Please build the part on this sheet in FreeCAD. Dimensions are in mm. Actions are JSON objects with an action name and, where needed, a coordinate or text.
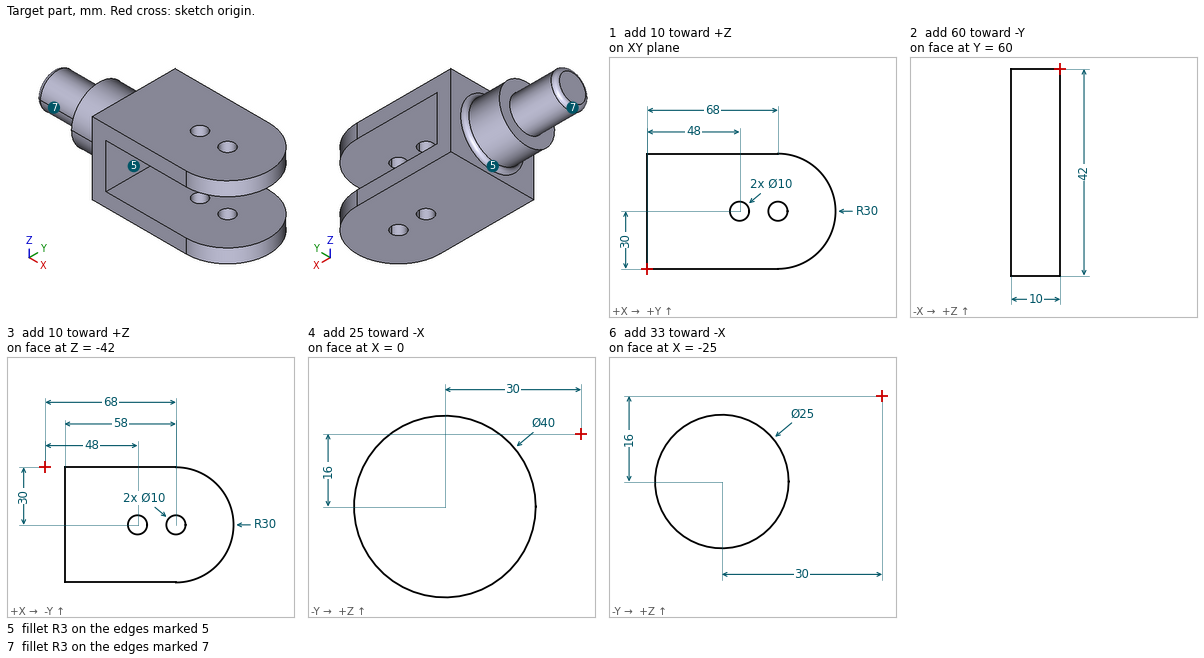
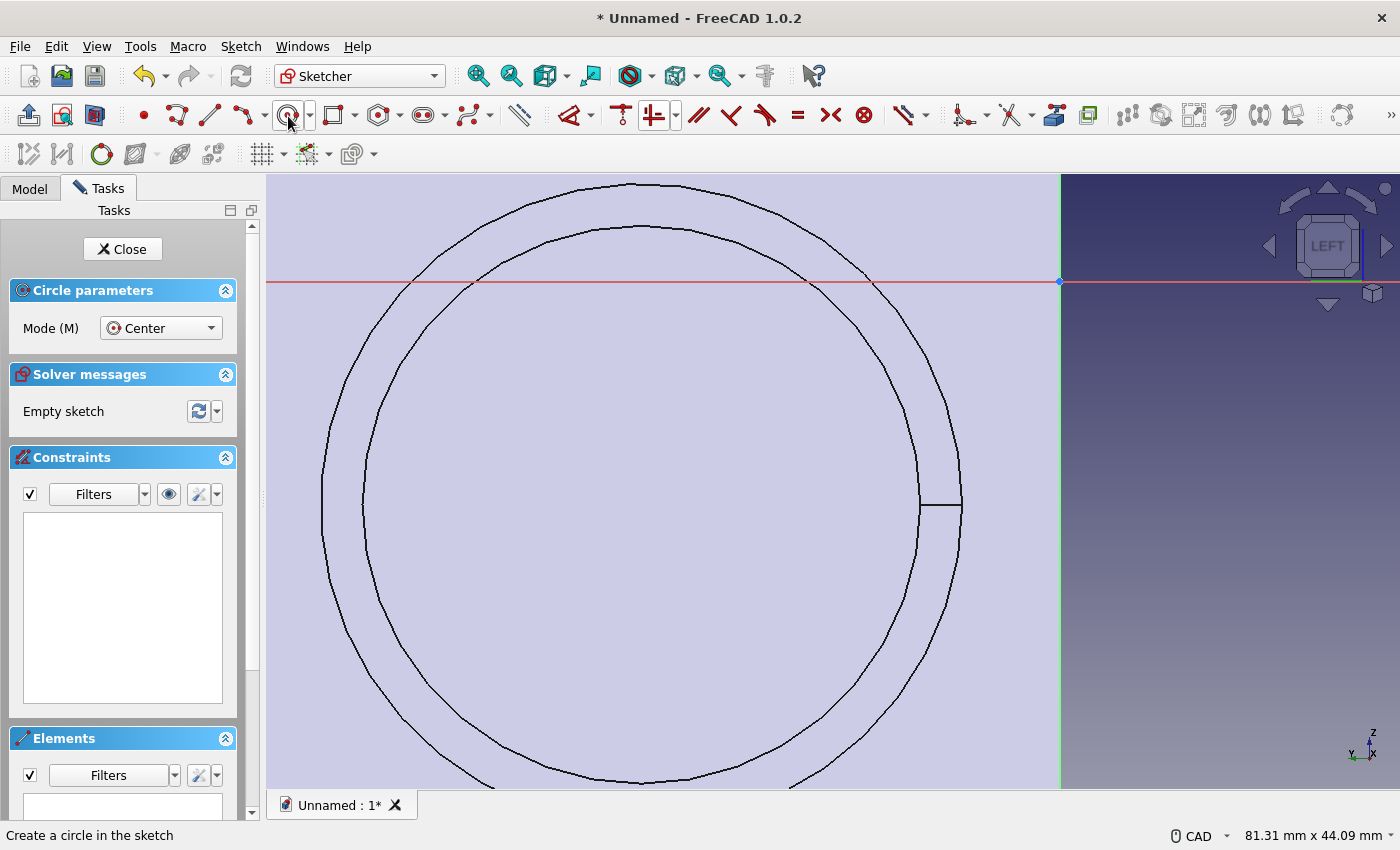
{"action": "left_click", "coordinate": [641, 505]}
{"action": "mouse_move", "coordinate": [765, 381]}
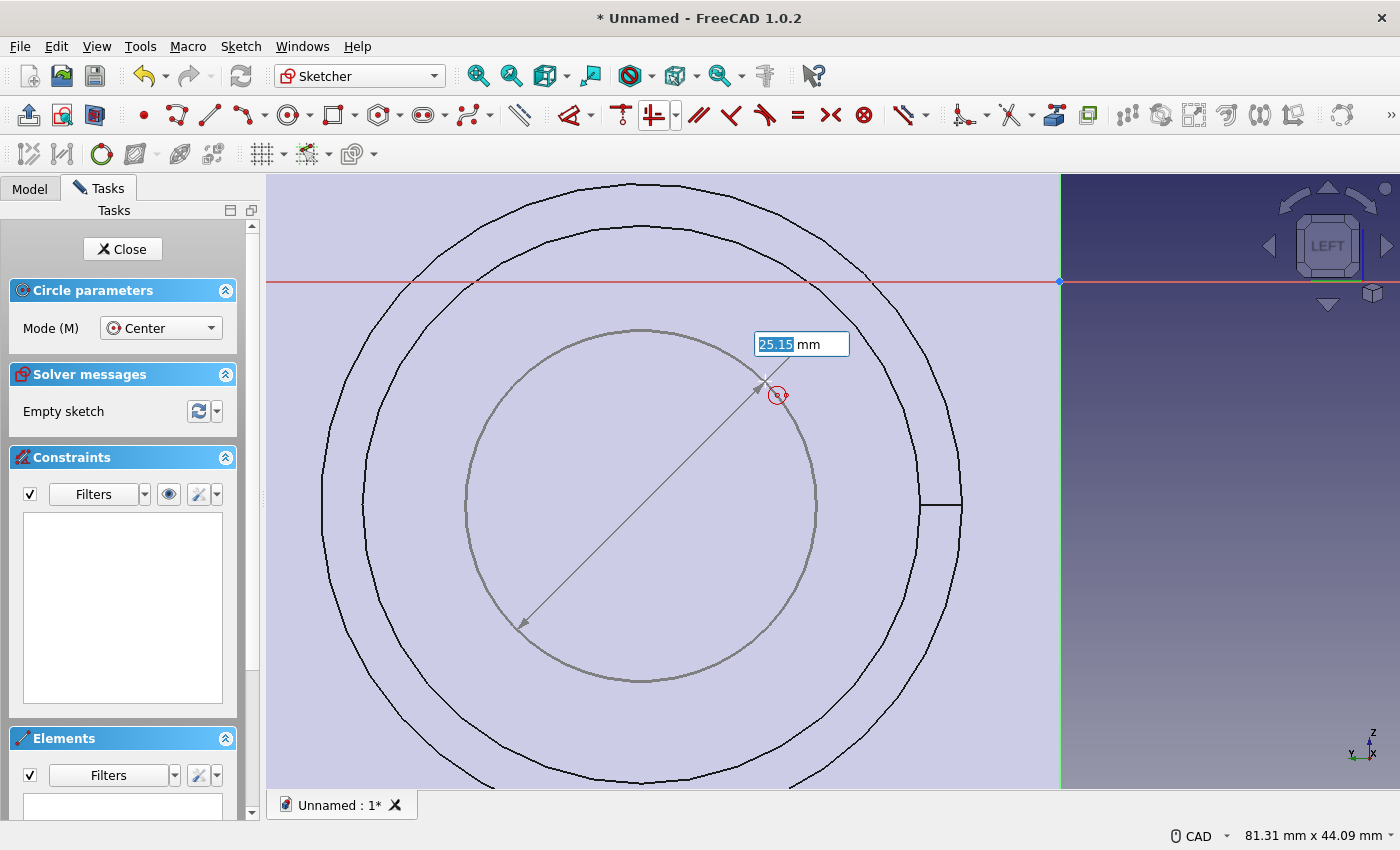
{"action": "type", "text": "25"}
{"action": "key", "text": "Return"}
{"action": "key", "text": "Escape"}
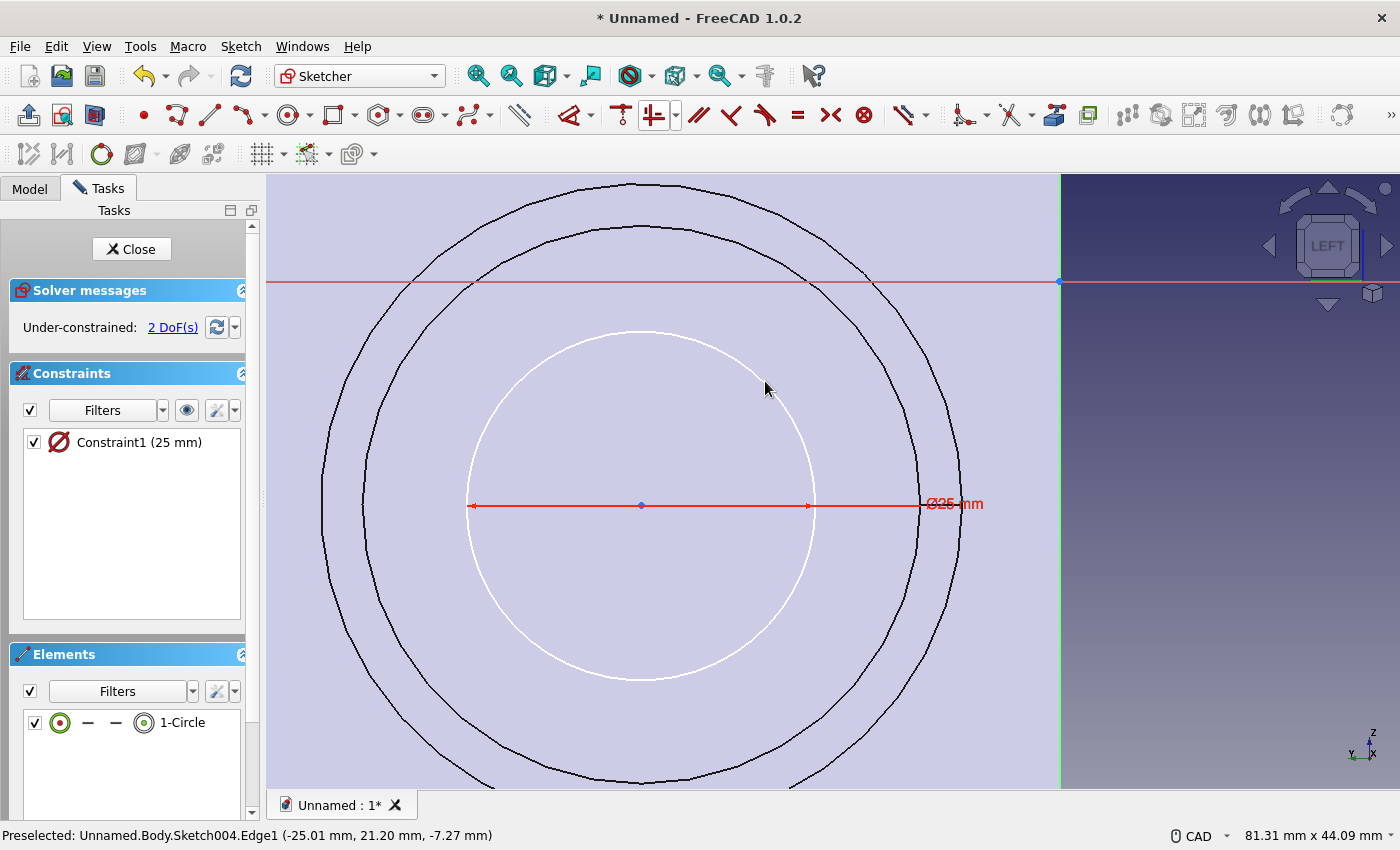
{"action": "left_click", "coordinate": [568, 116]}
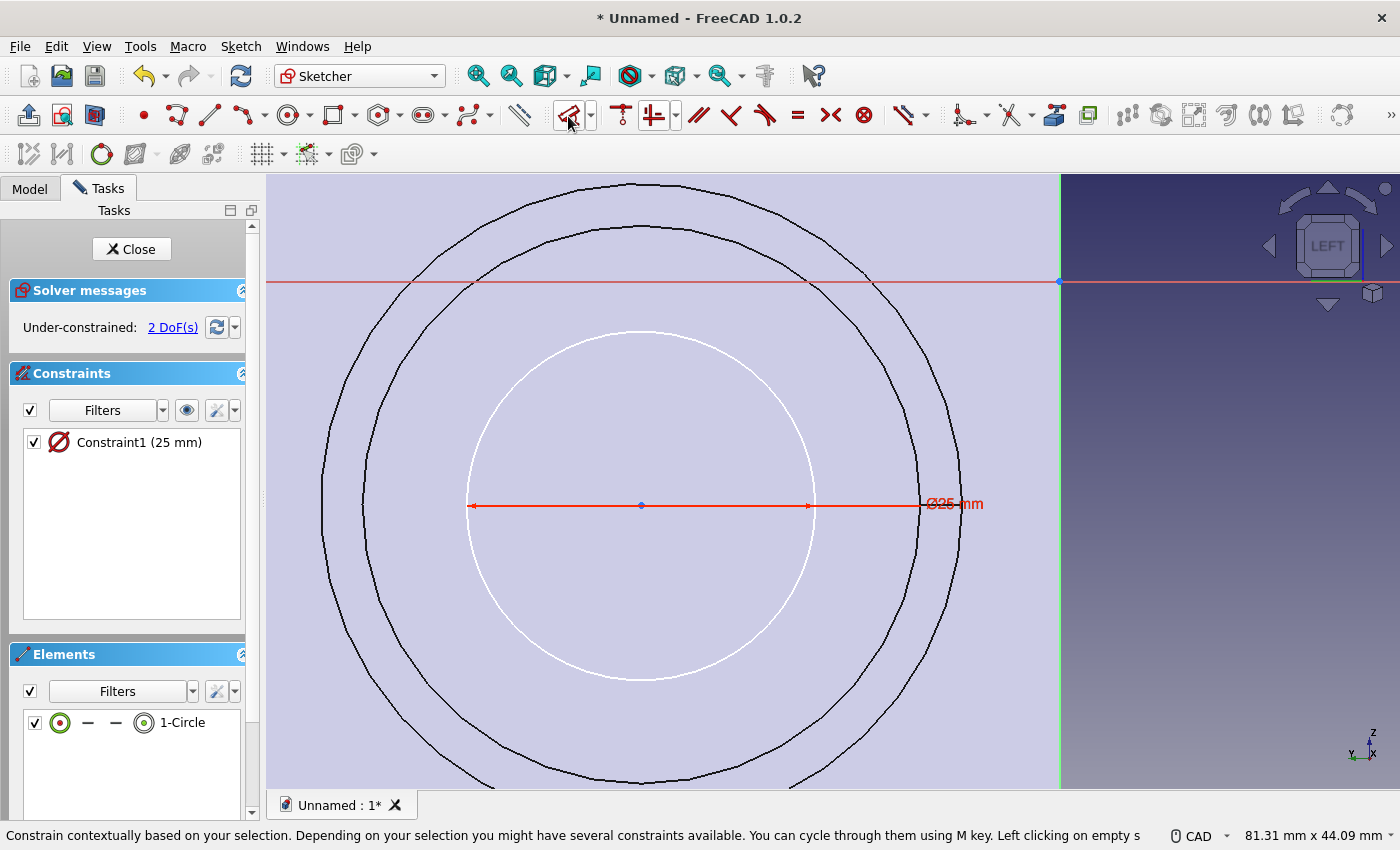
{"action": "left_click", "coordinate": [641, 506]}
{"action": "left_click", "coordinate": [850, 248]}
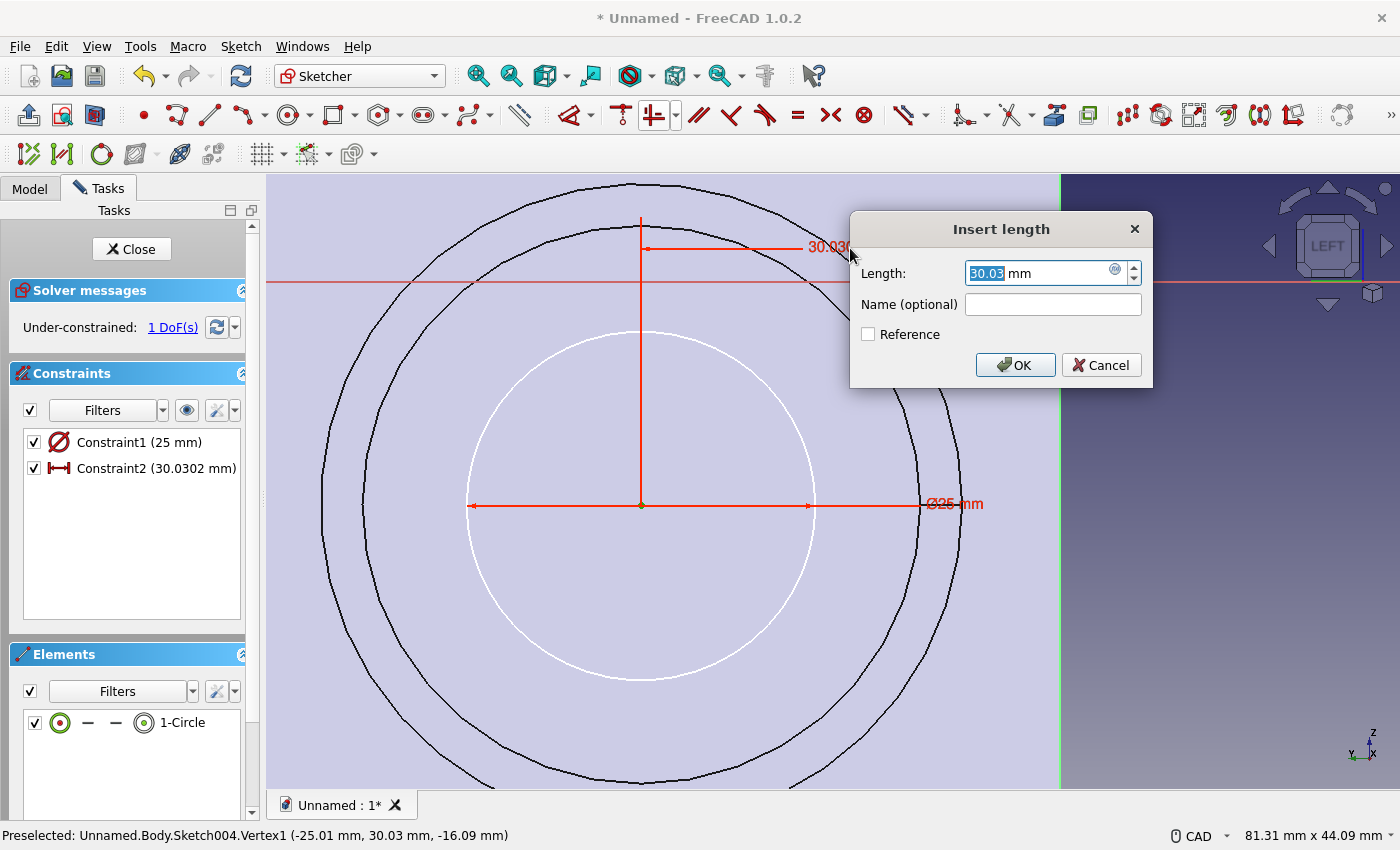
{"action": "type", "text": "30"}
{"action": "key", "text": "Return"}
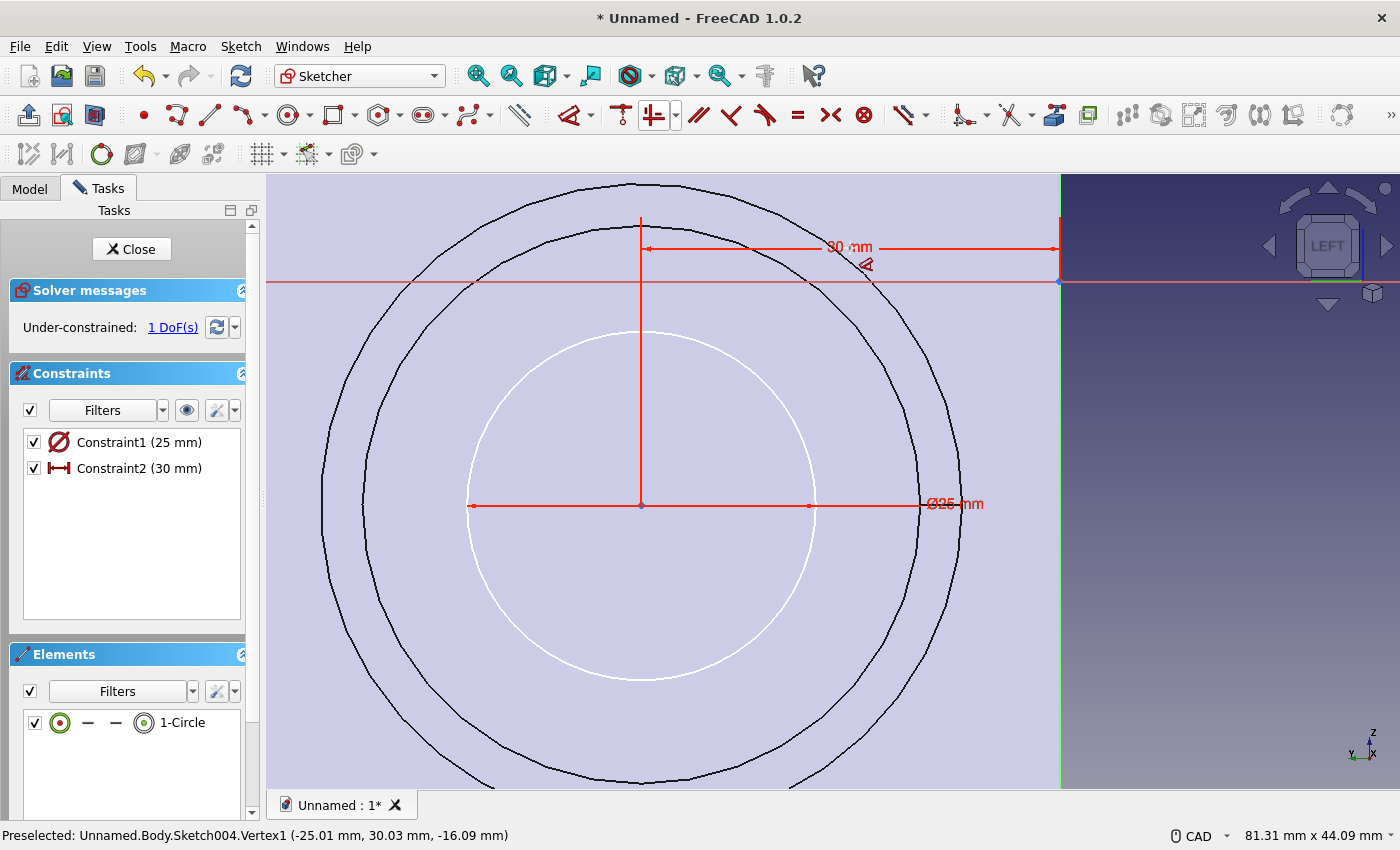
{"action": "left_click", "coordinate": [641, 506]}
{"action": "left_click", "coordinate": [1094, 394]}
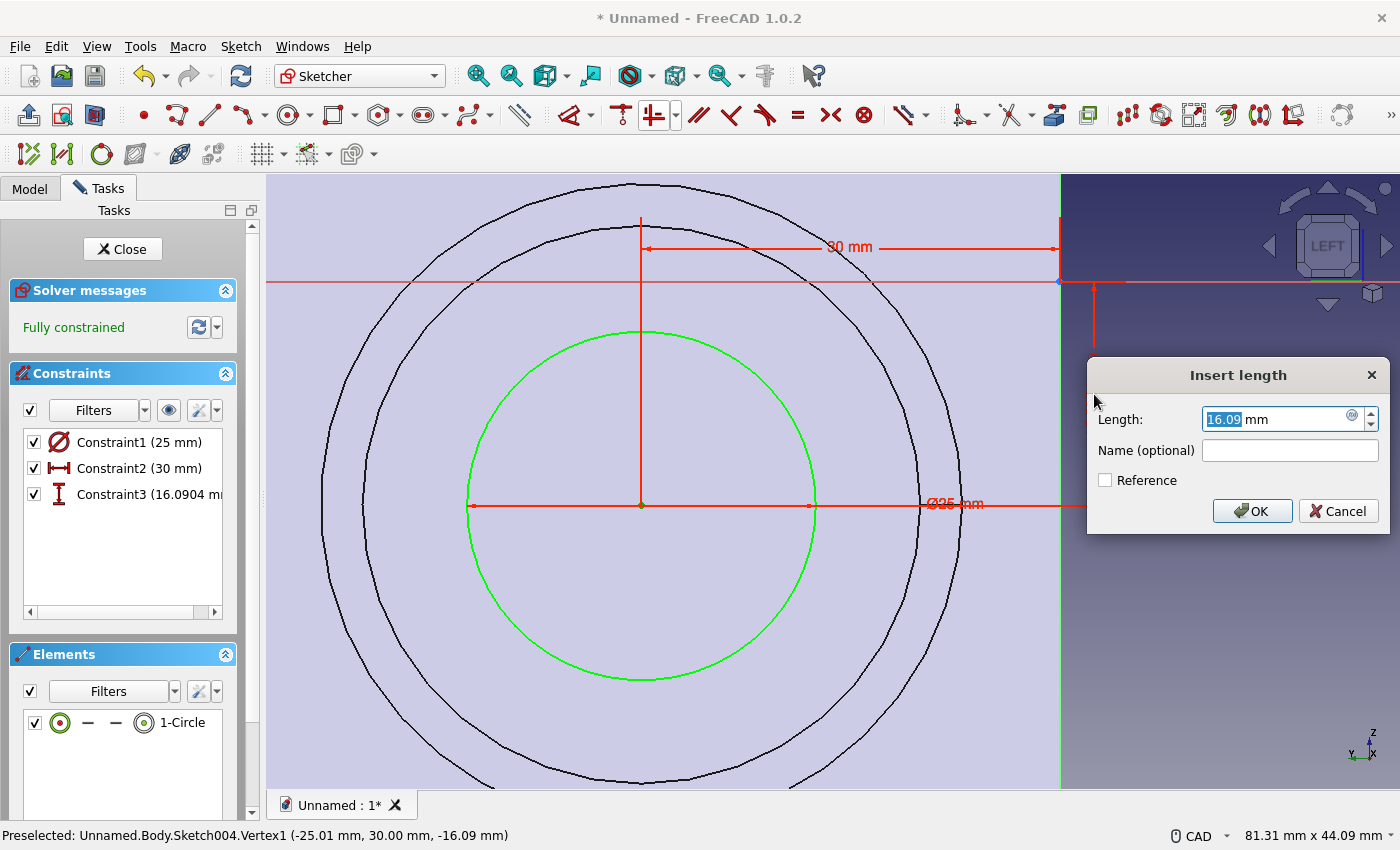
{"action": "type", "text": "16"}
{"action": "key", "text": "Return"}
{"action": "key", "text": "Escape"}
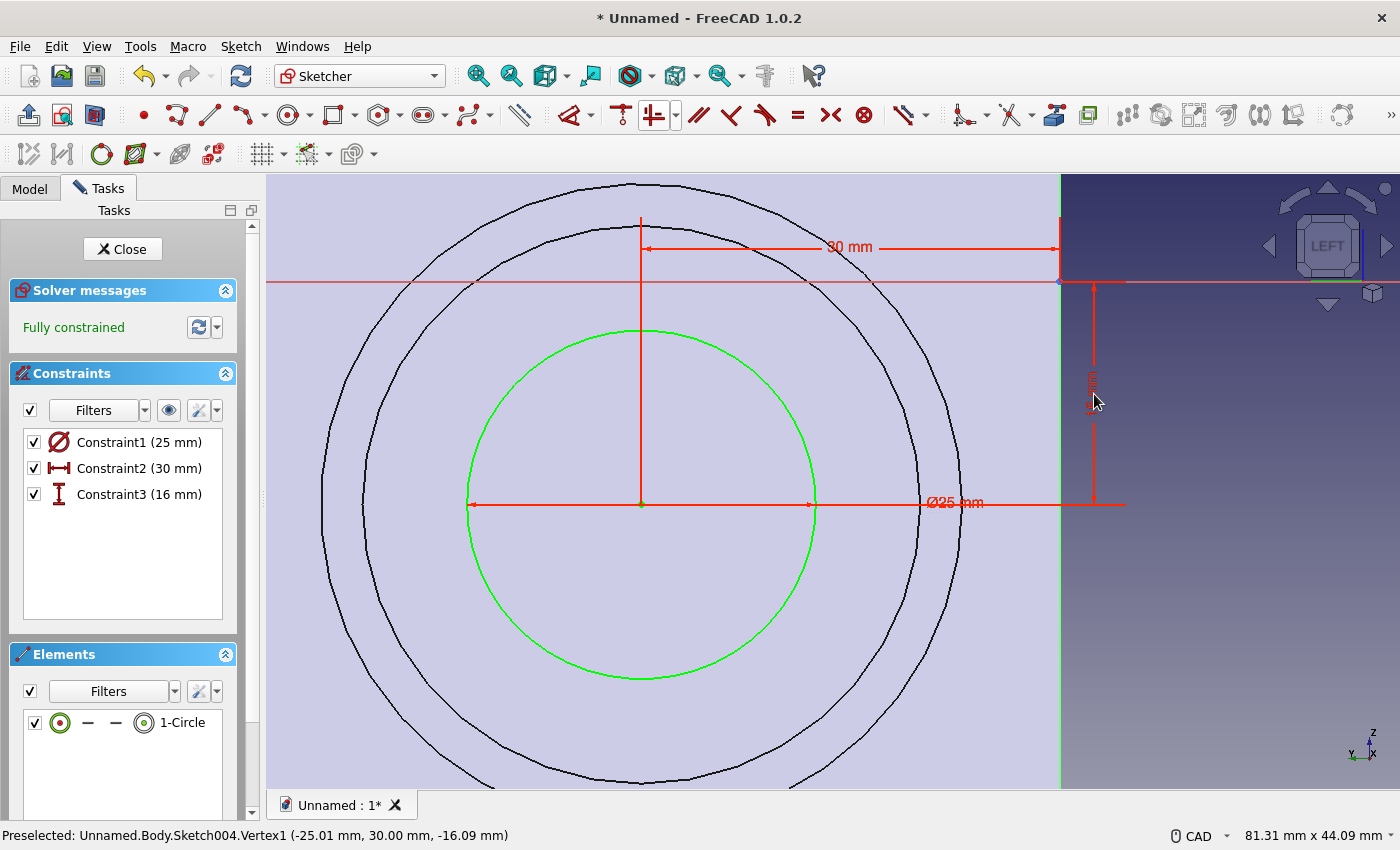
{"action": "left_click", "coordinate": [123, 249]}